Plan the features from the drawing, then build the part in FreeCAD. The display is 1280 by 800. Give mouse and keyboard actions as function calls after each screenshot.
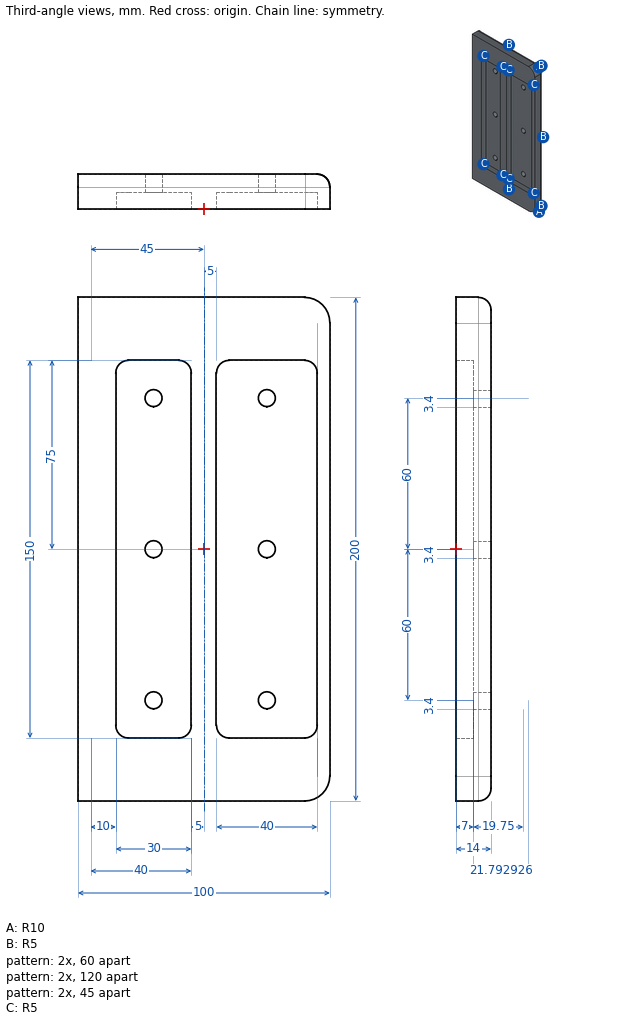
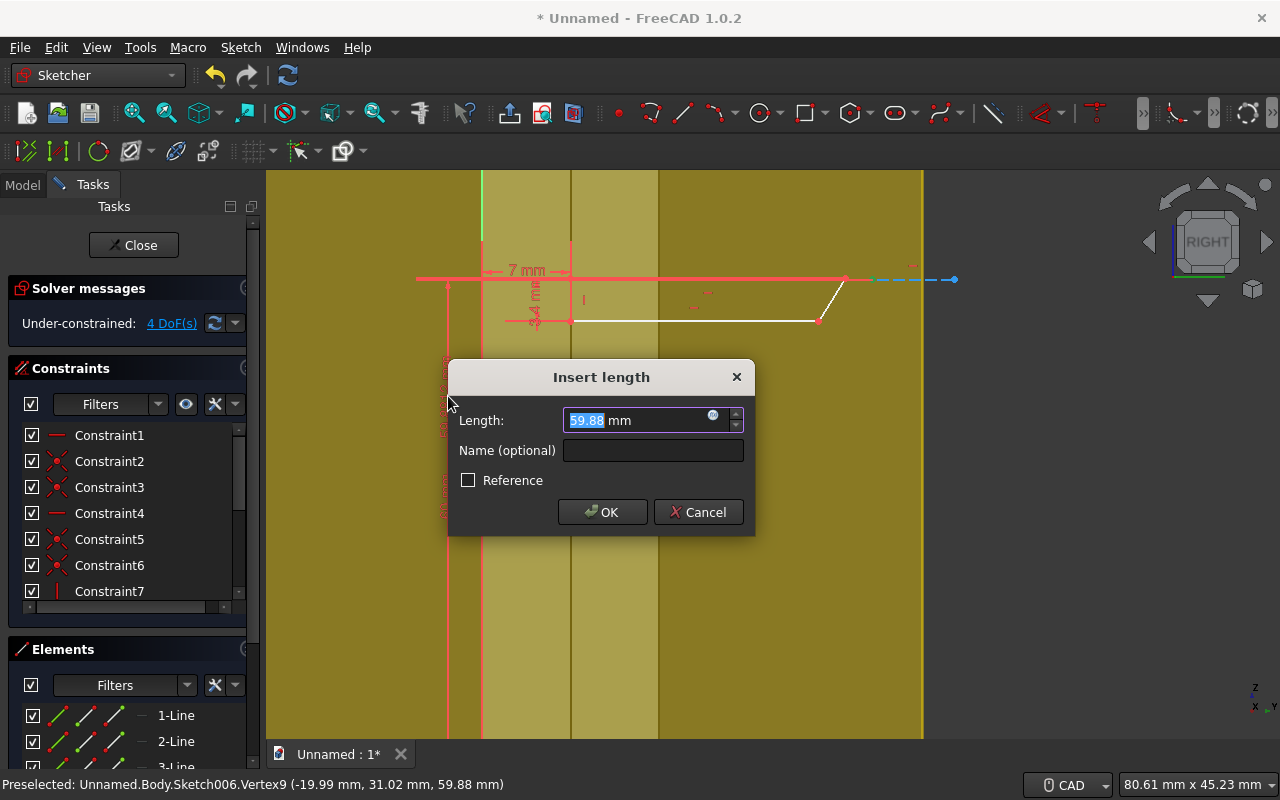
text(60)
key(Return)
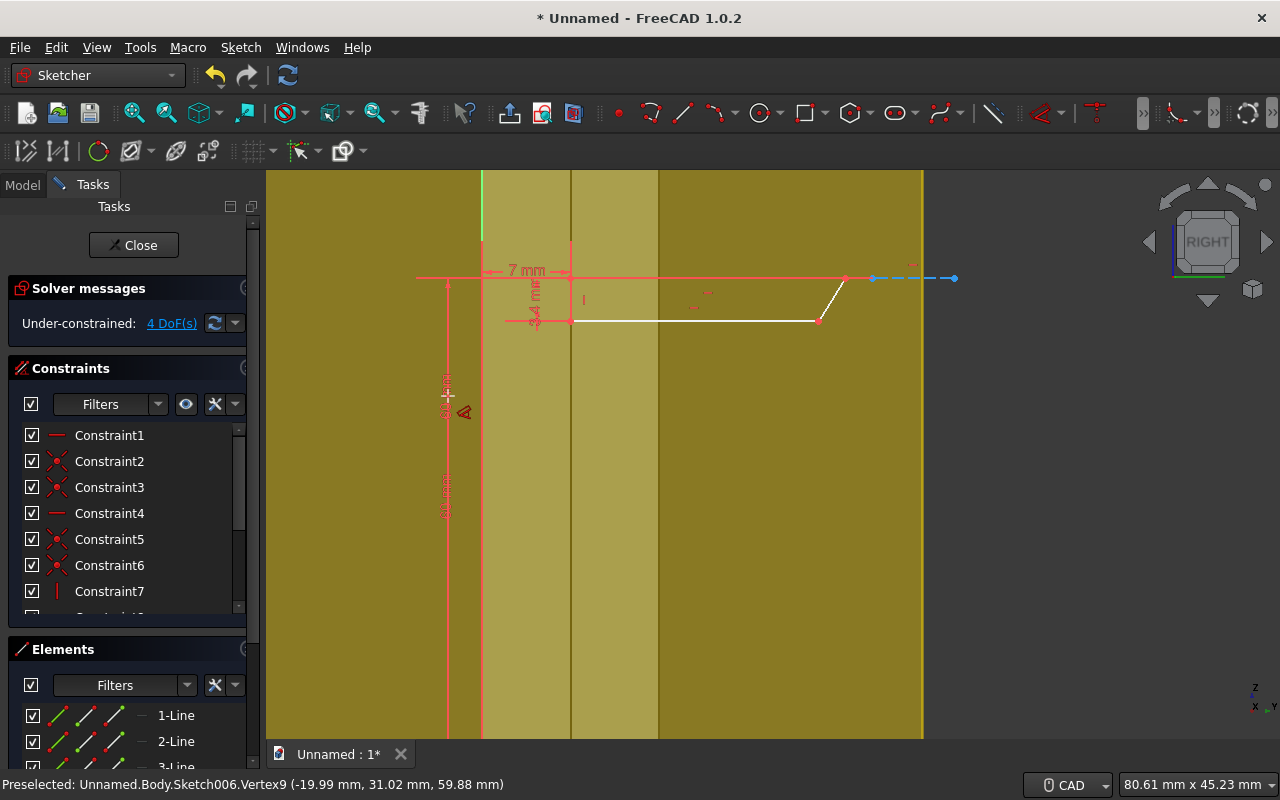
click(645, 321)
click(695, 355)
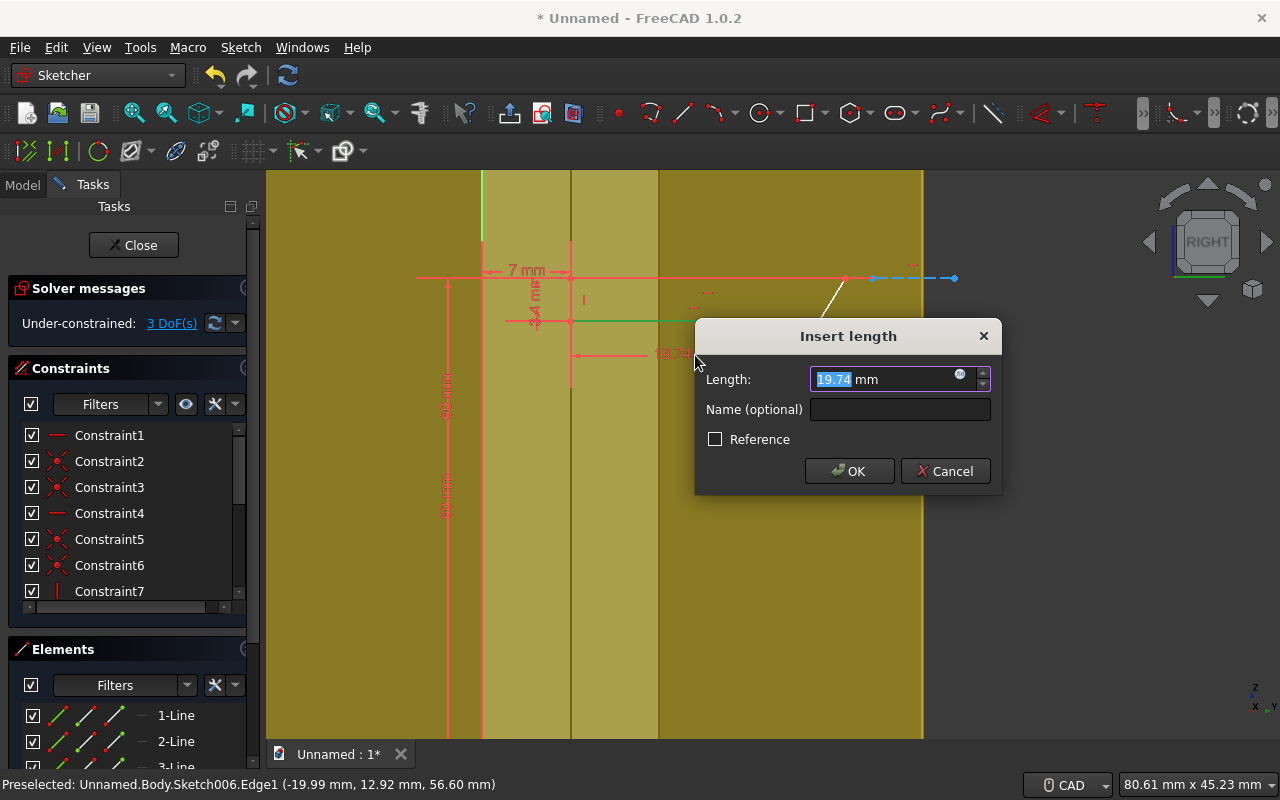
text(19.75)
key(Return)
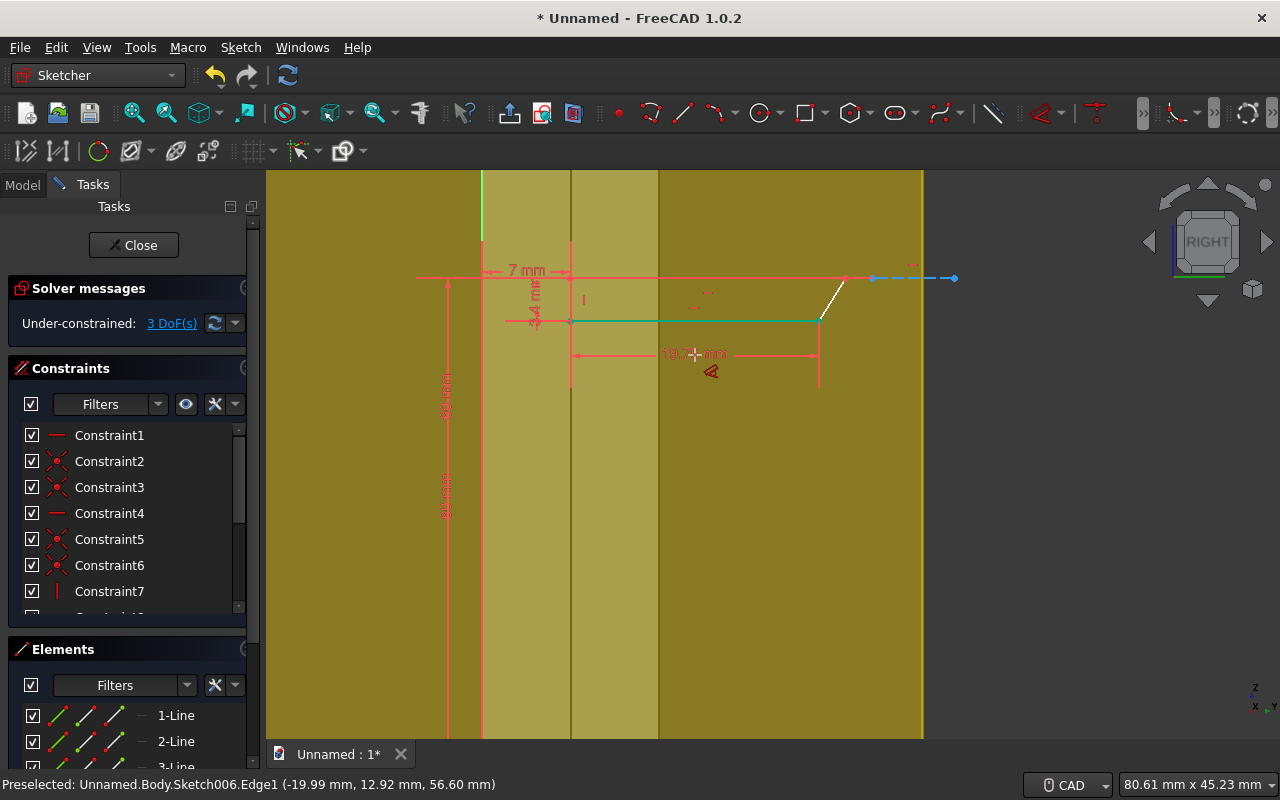
click(763, 278)
click(708, 244)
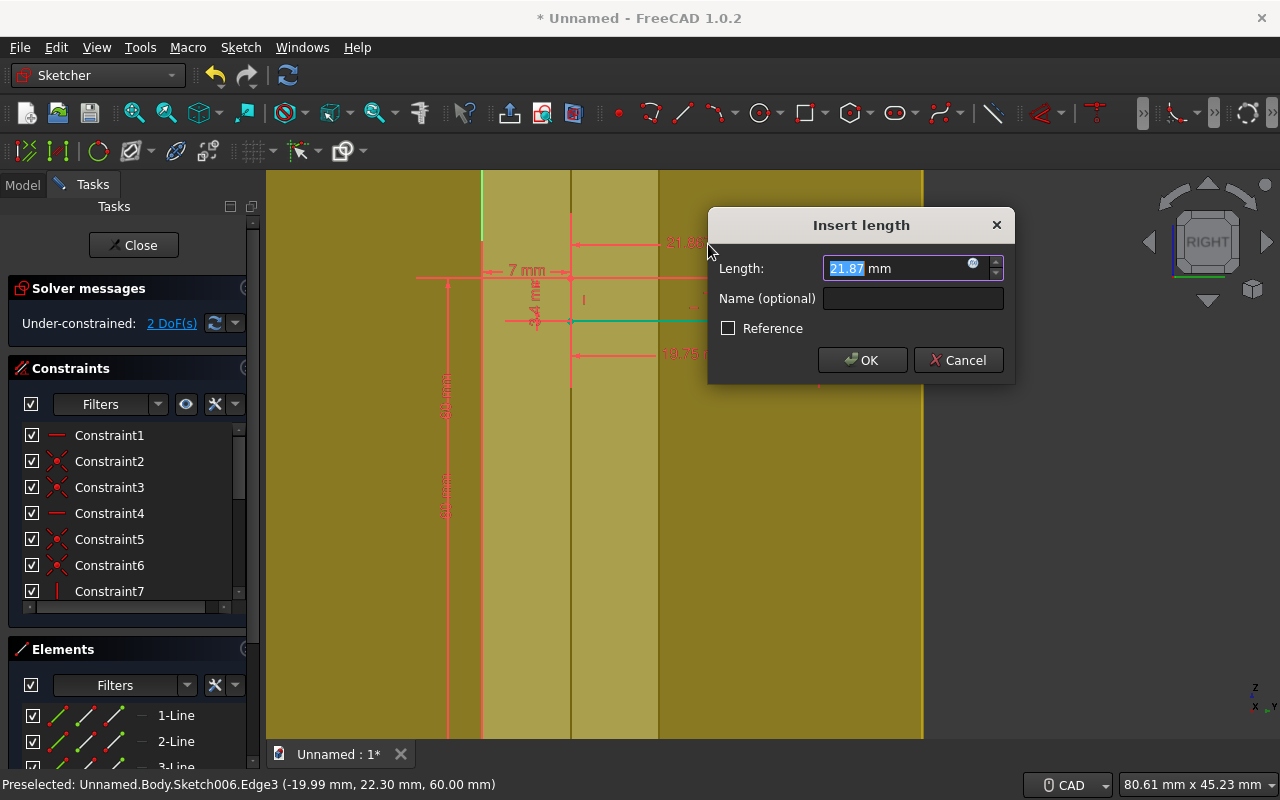
text(21.792926)
key(Return)
key(Escape)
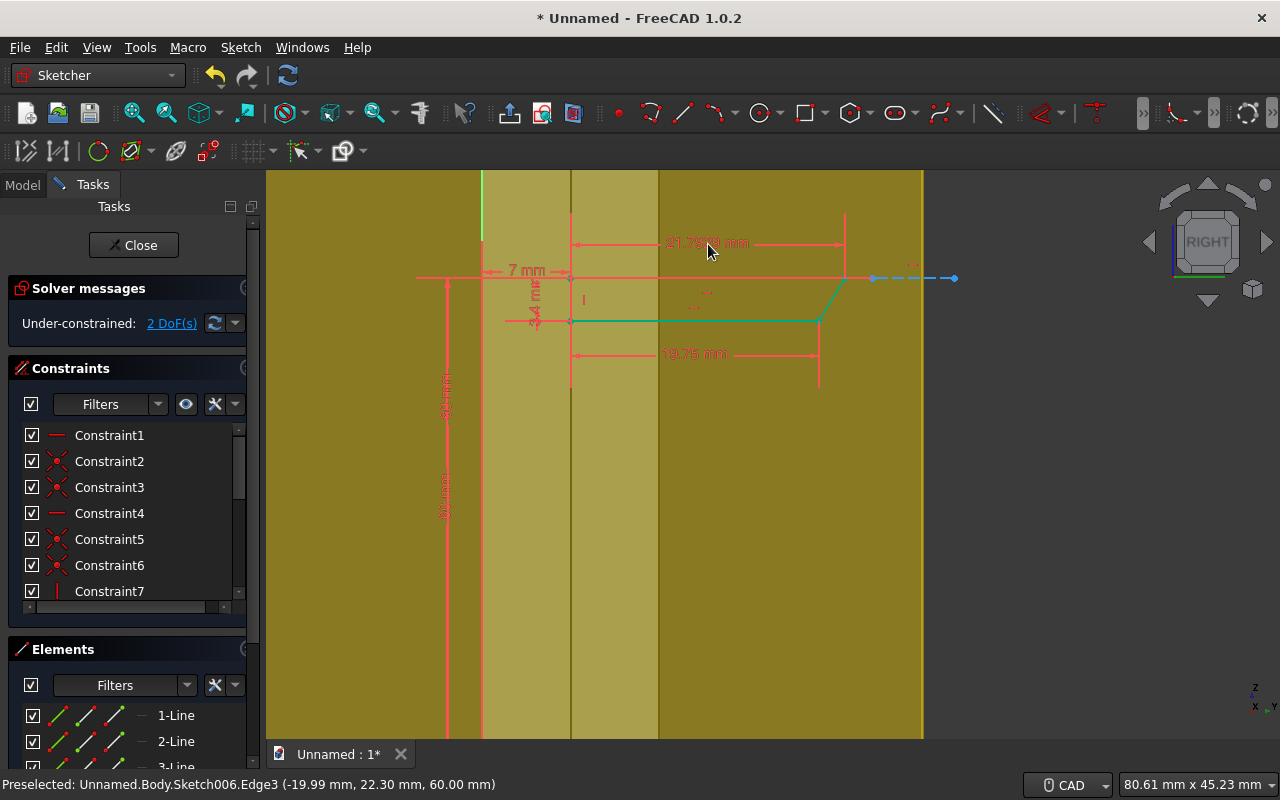
click(134, 245)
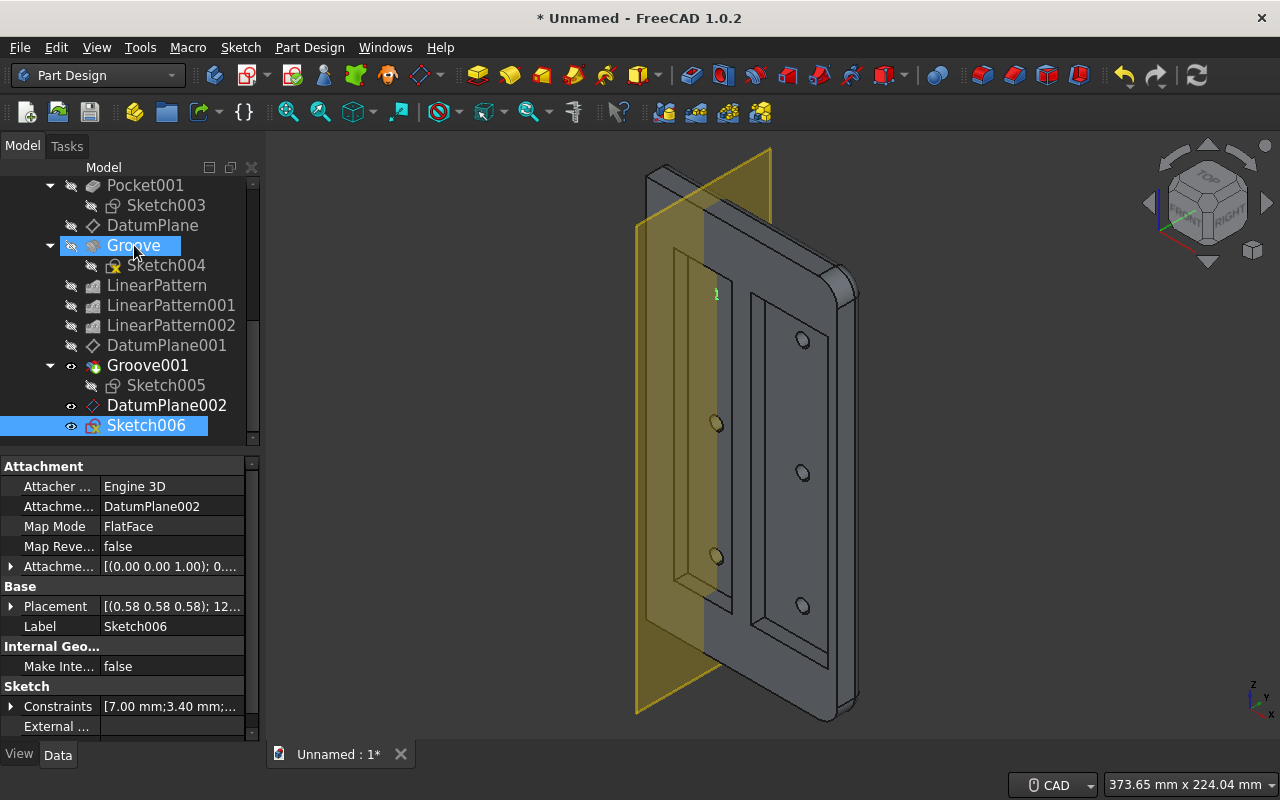
click(756, 76)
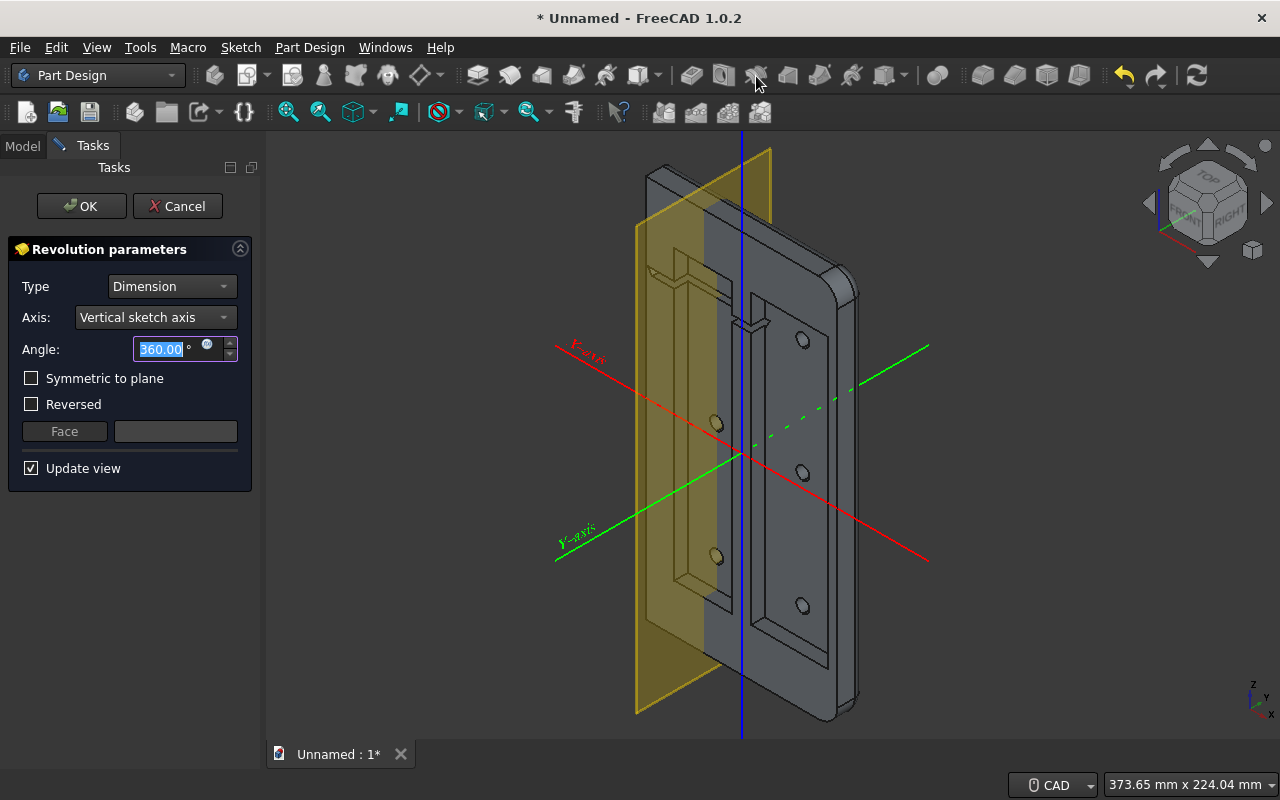
click(156, 318)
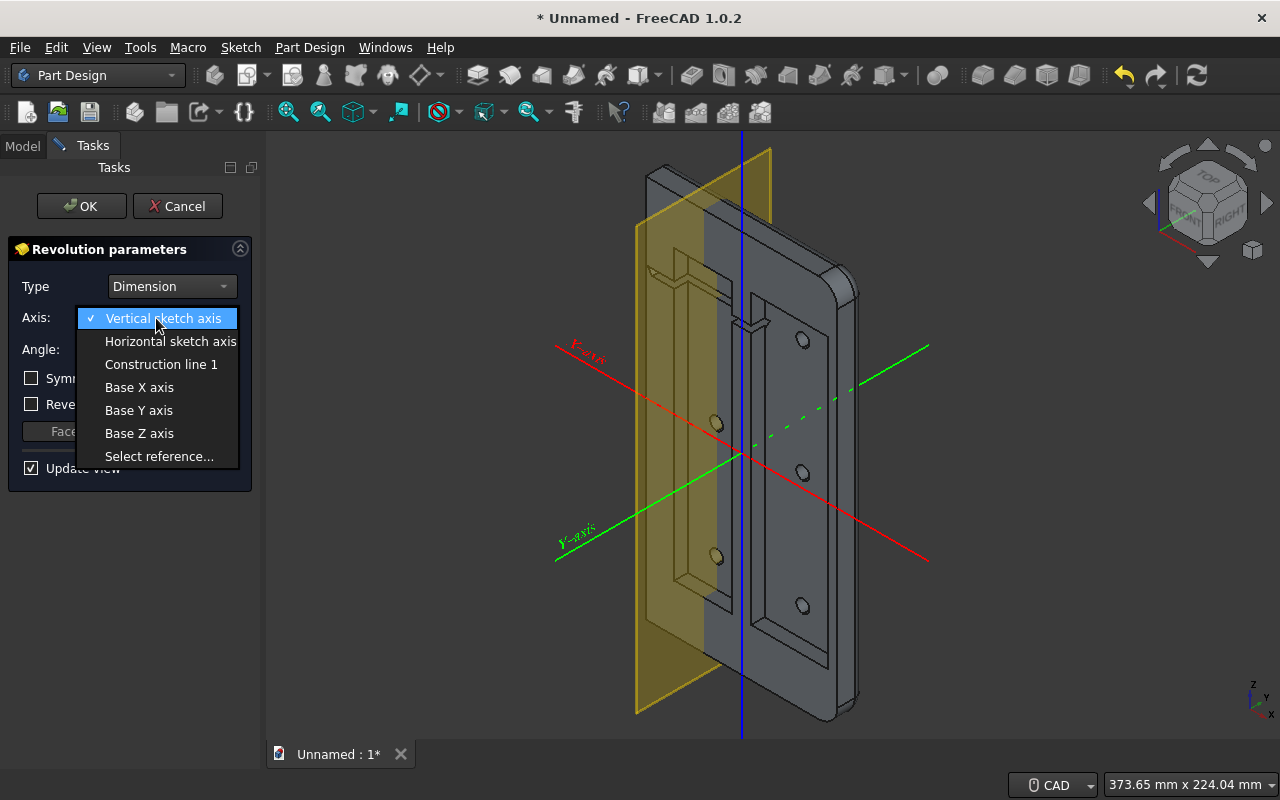
click(156, 364)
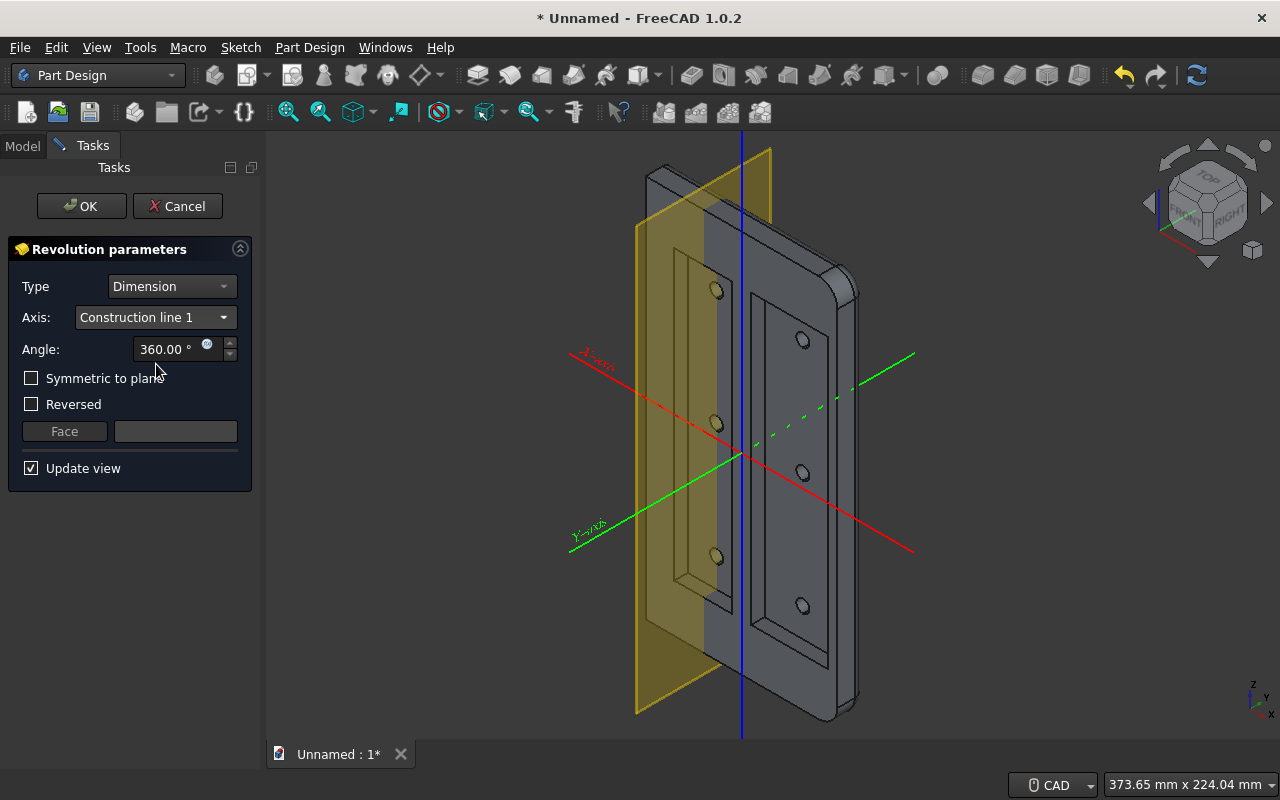
click(82, 206)